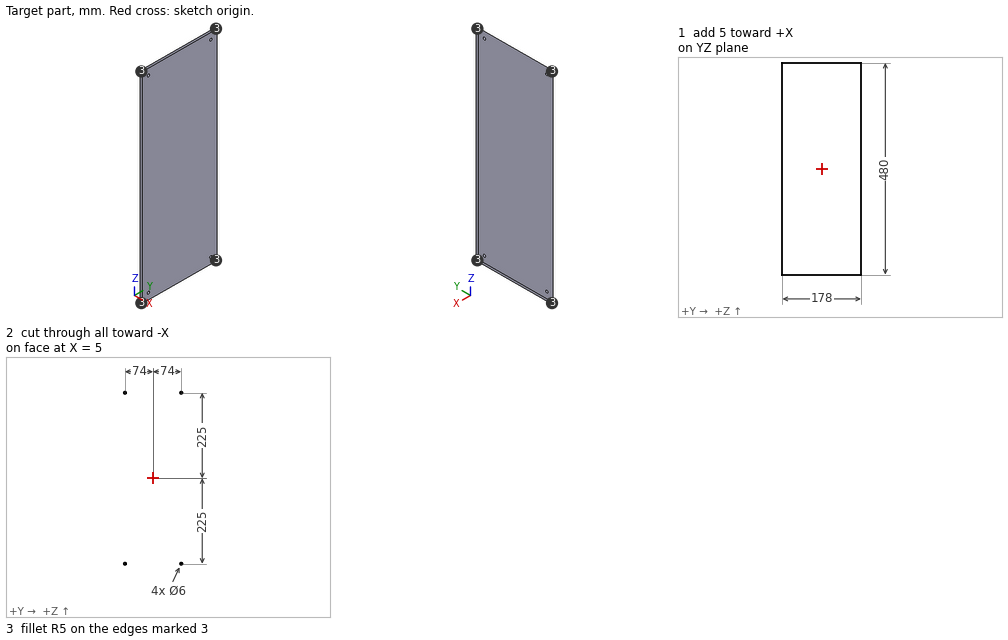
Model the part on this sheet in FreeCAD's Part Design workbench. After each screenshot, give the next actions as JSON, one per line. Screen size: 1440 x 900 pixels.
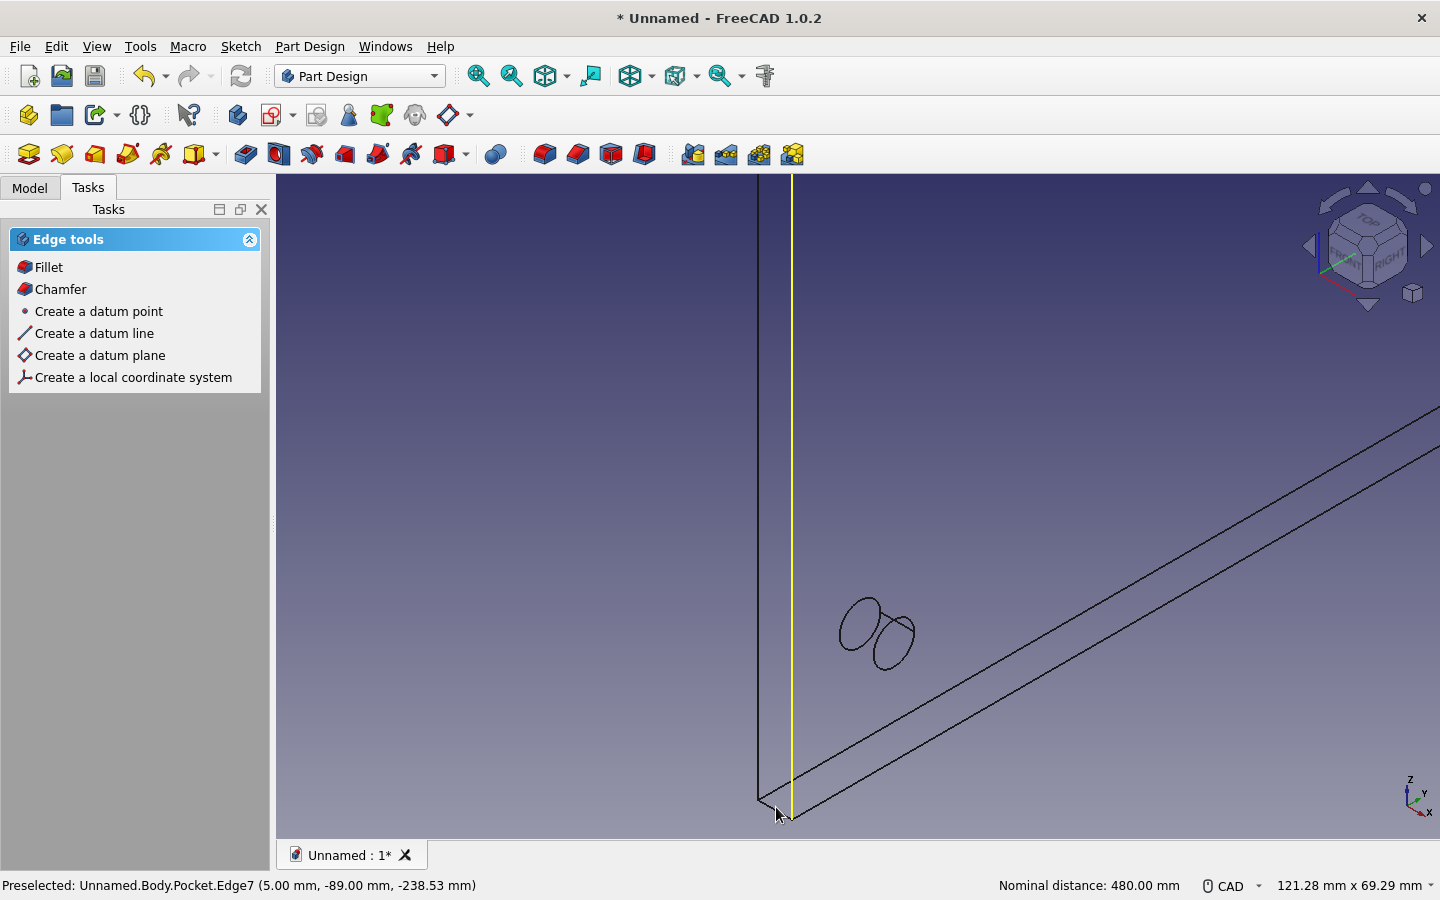
{"action": "left_click", "coordinate": [775, 809], "text": "ctrl"}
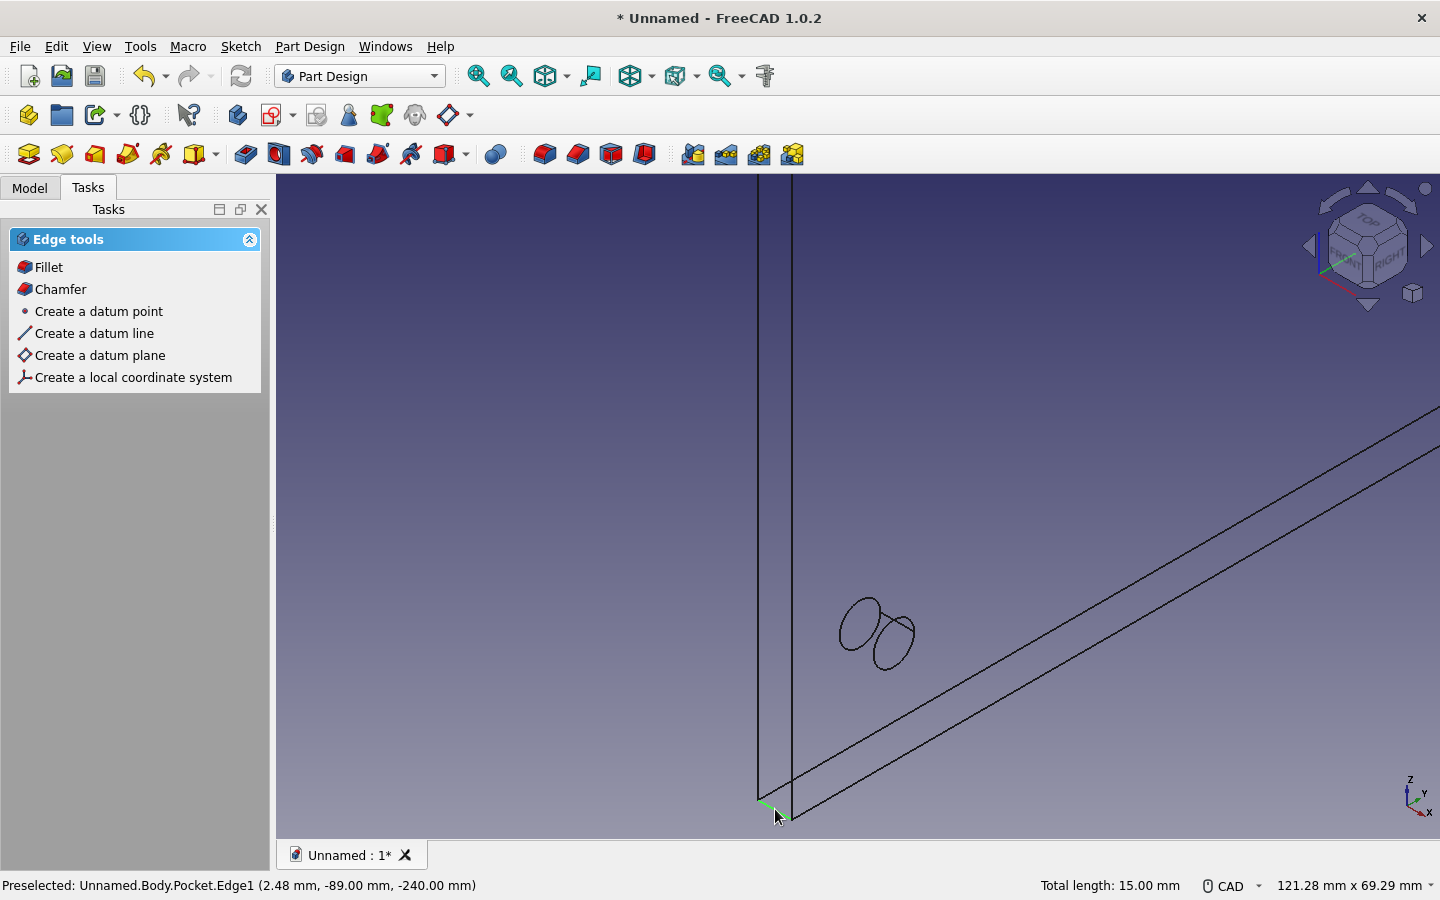
{"action": "left_click", "coordinate": [479, 76]}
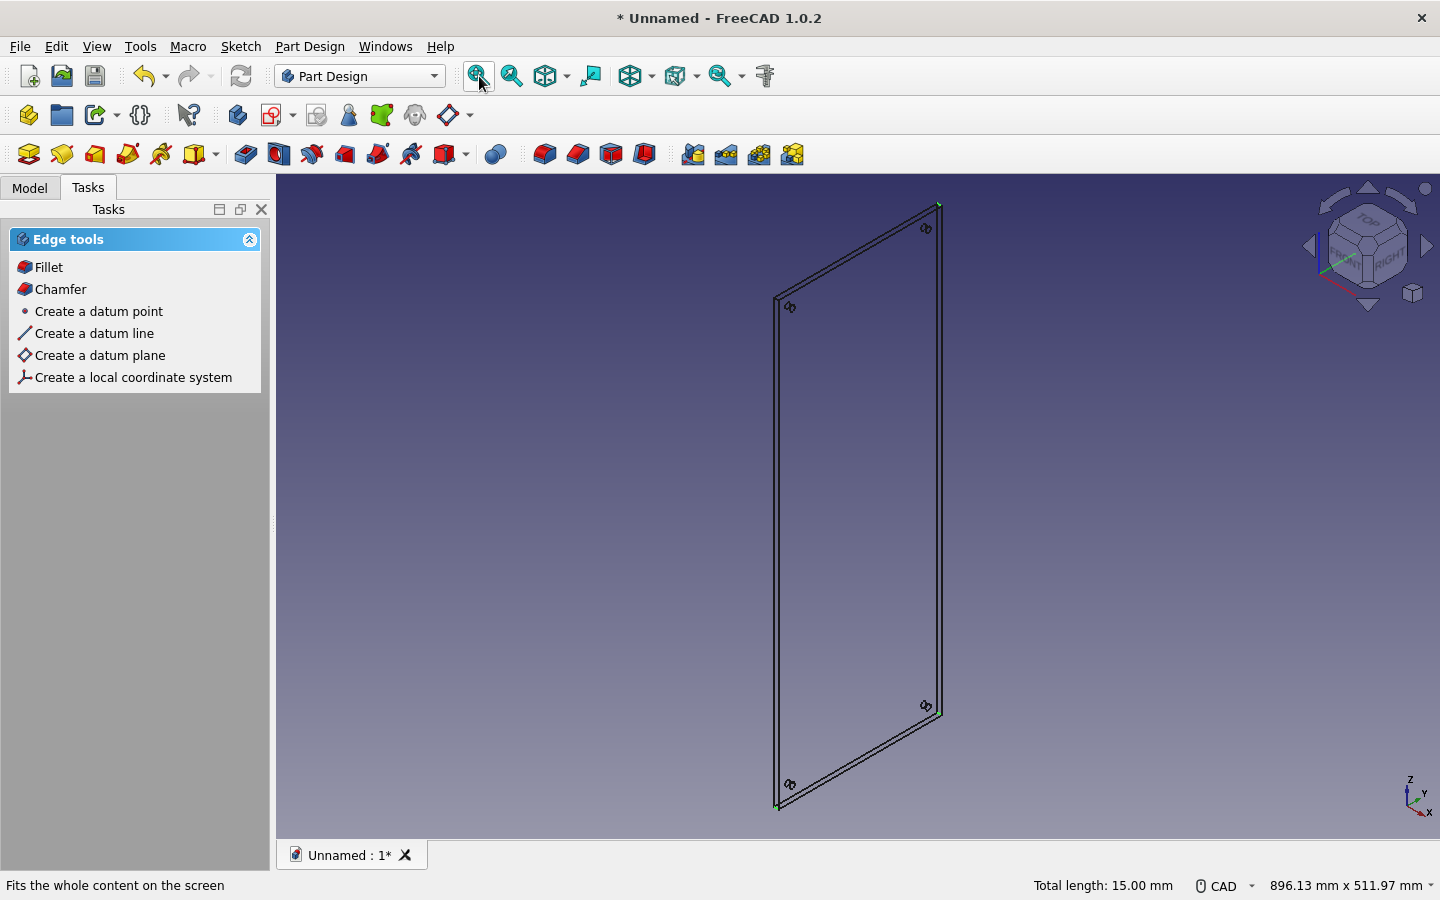
{"action": "key", "text": "2"}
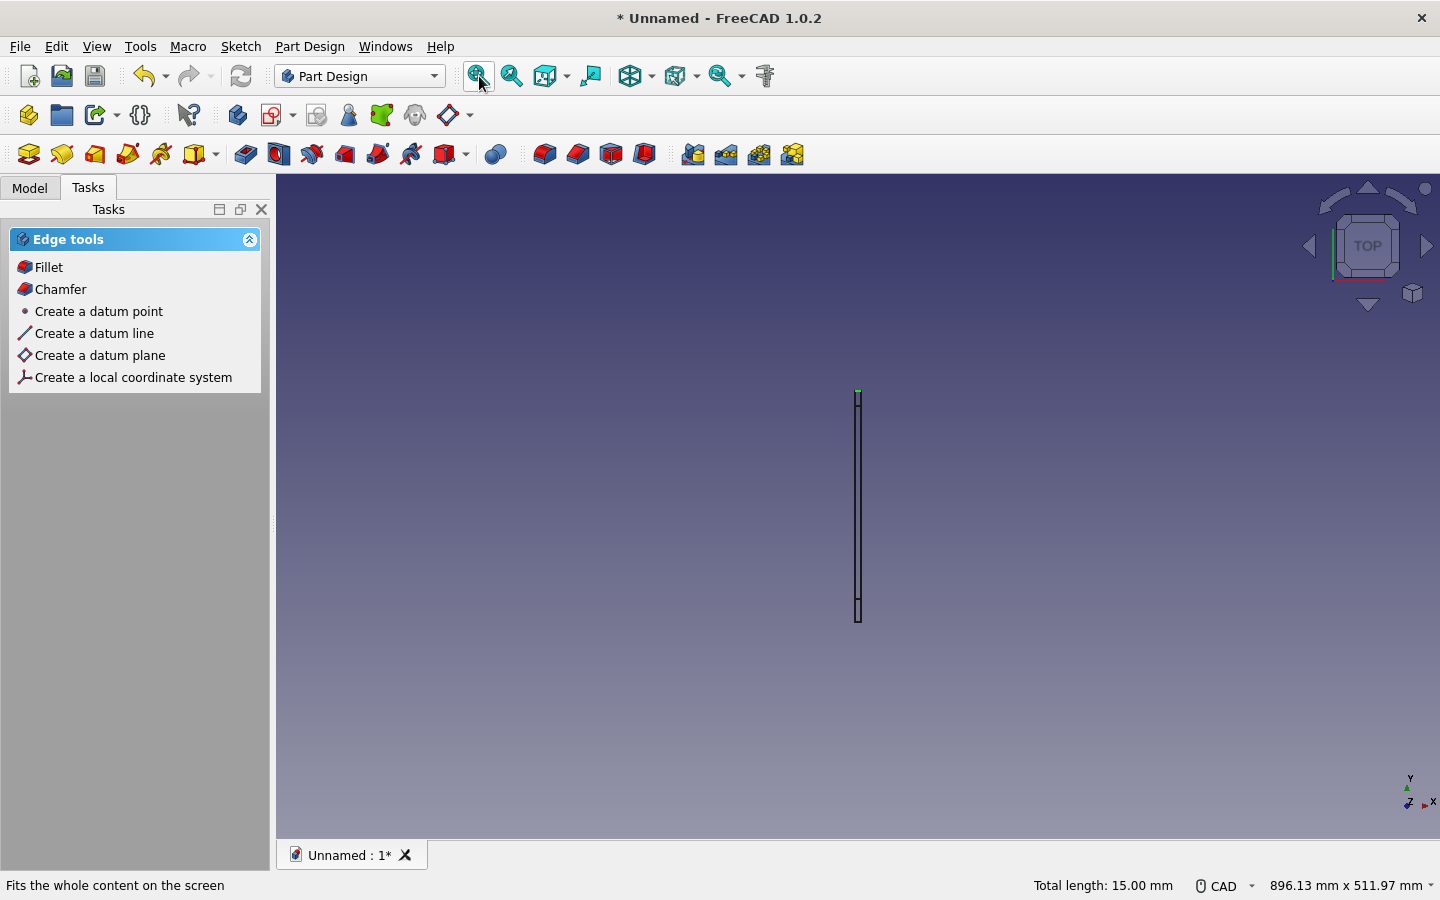
{"action": "left_click", "coordinate": [479, 76]}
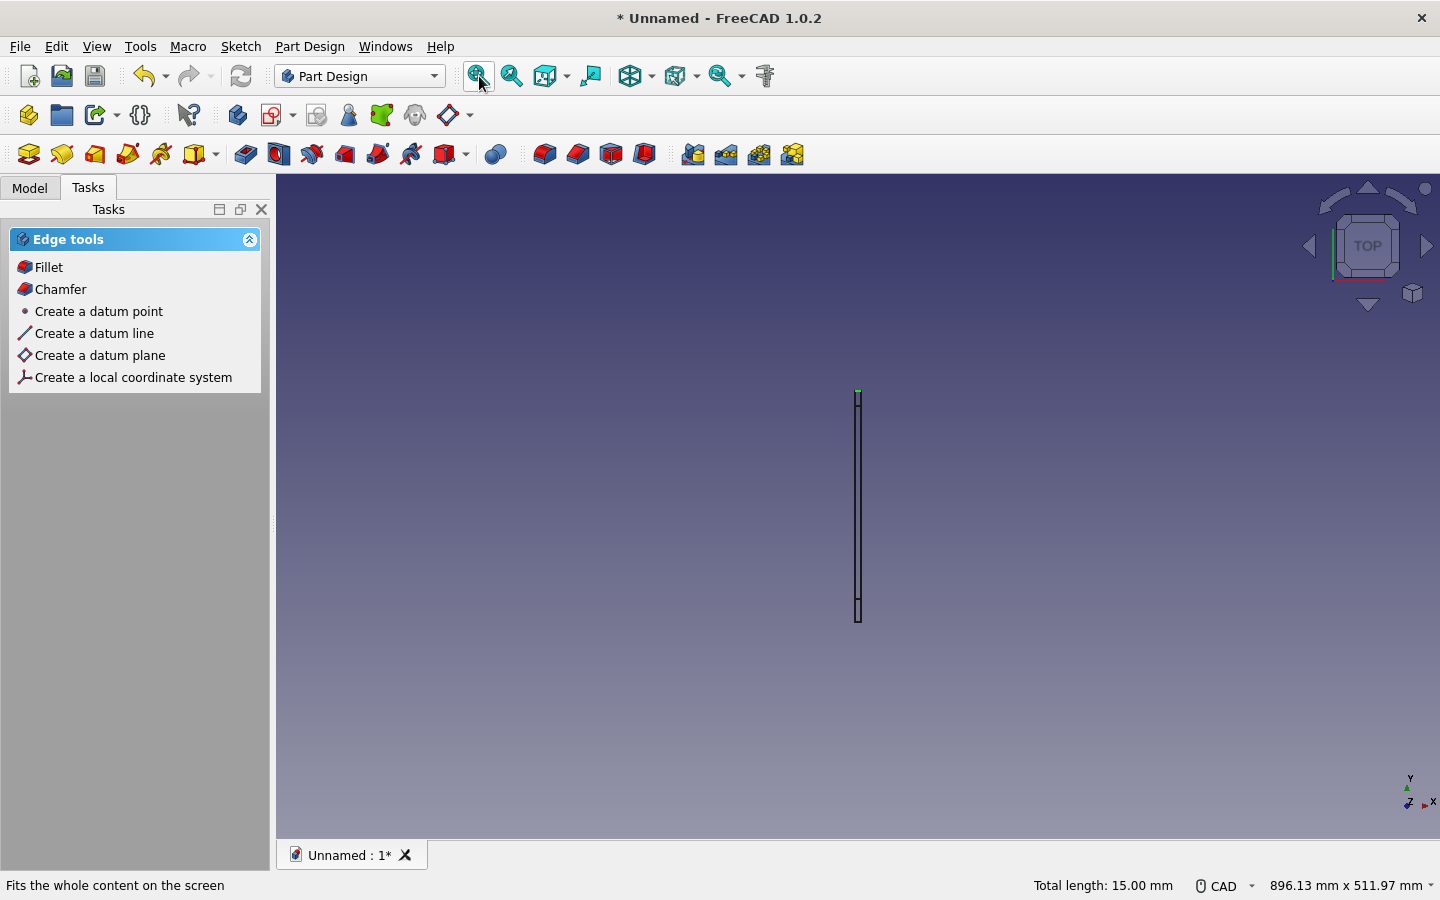
{"action": "scroll", "coordinate": [858, 621], "scroll_direction": "up", "scroll_amount": 10}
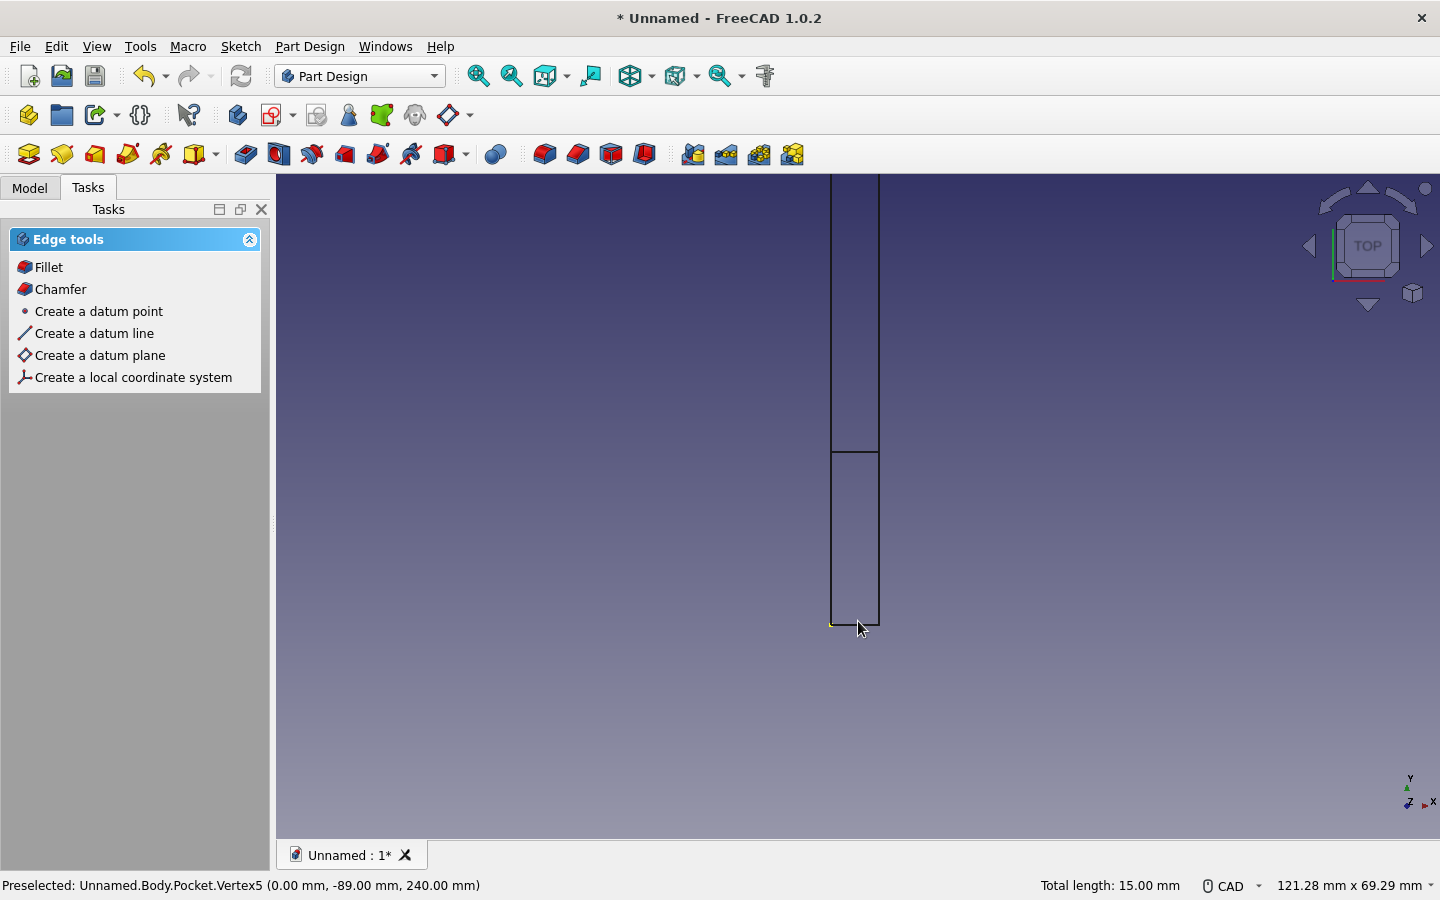
{"action": "left_click", "coordinate": [855, 624], "text": "ctrl"}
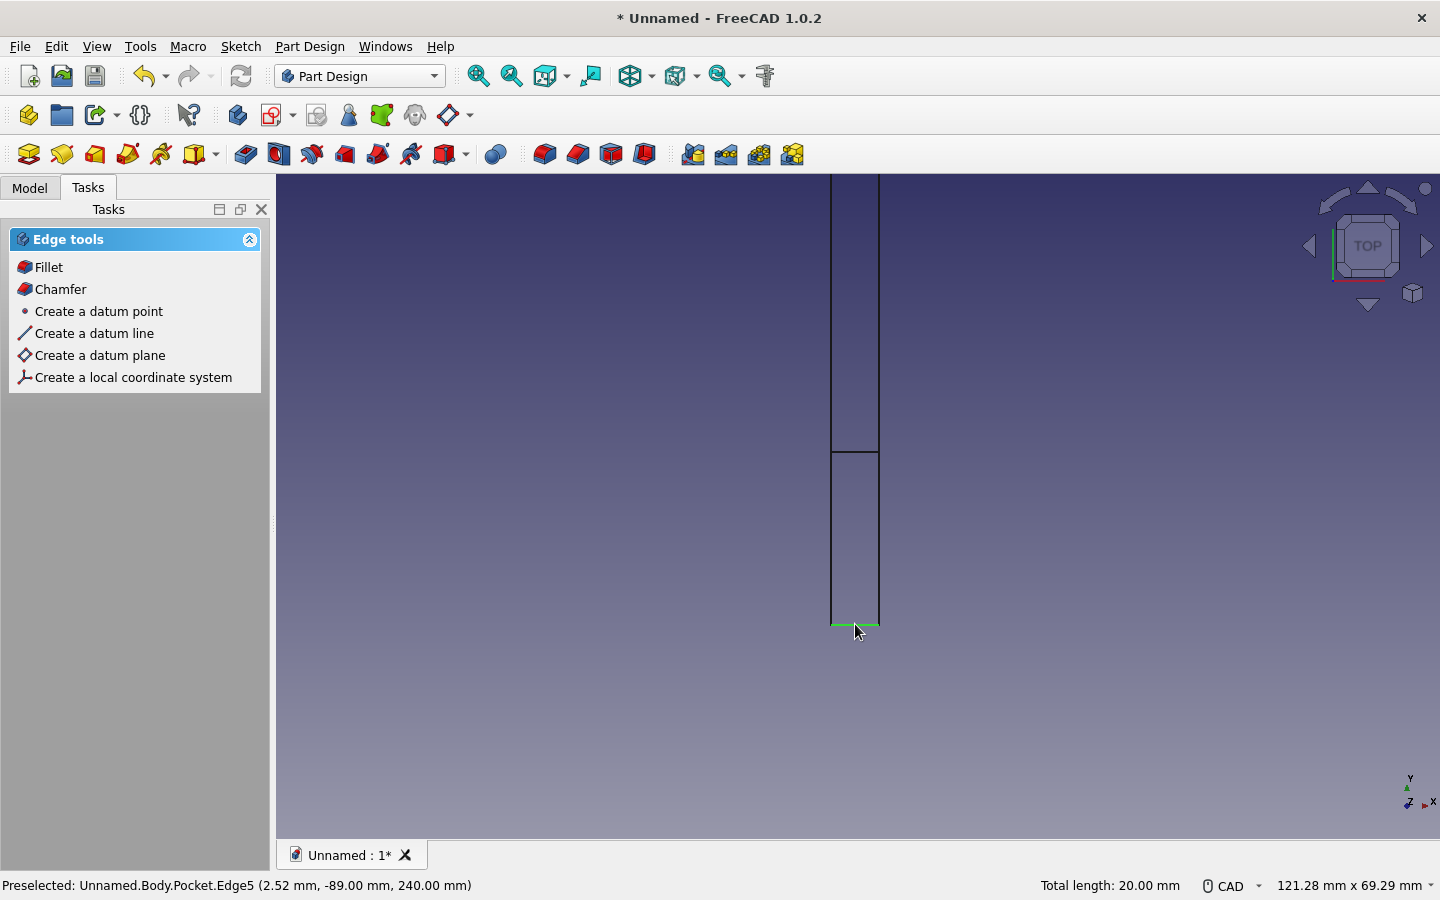
{"action": "key", "text": "v 1"}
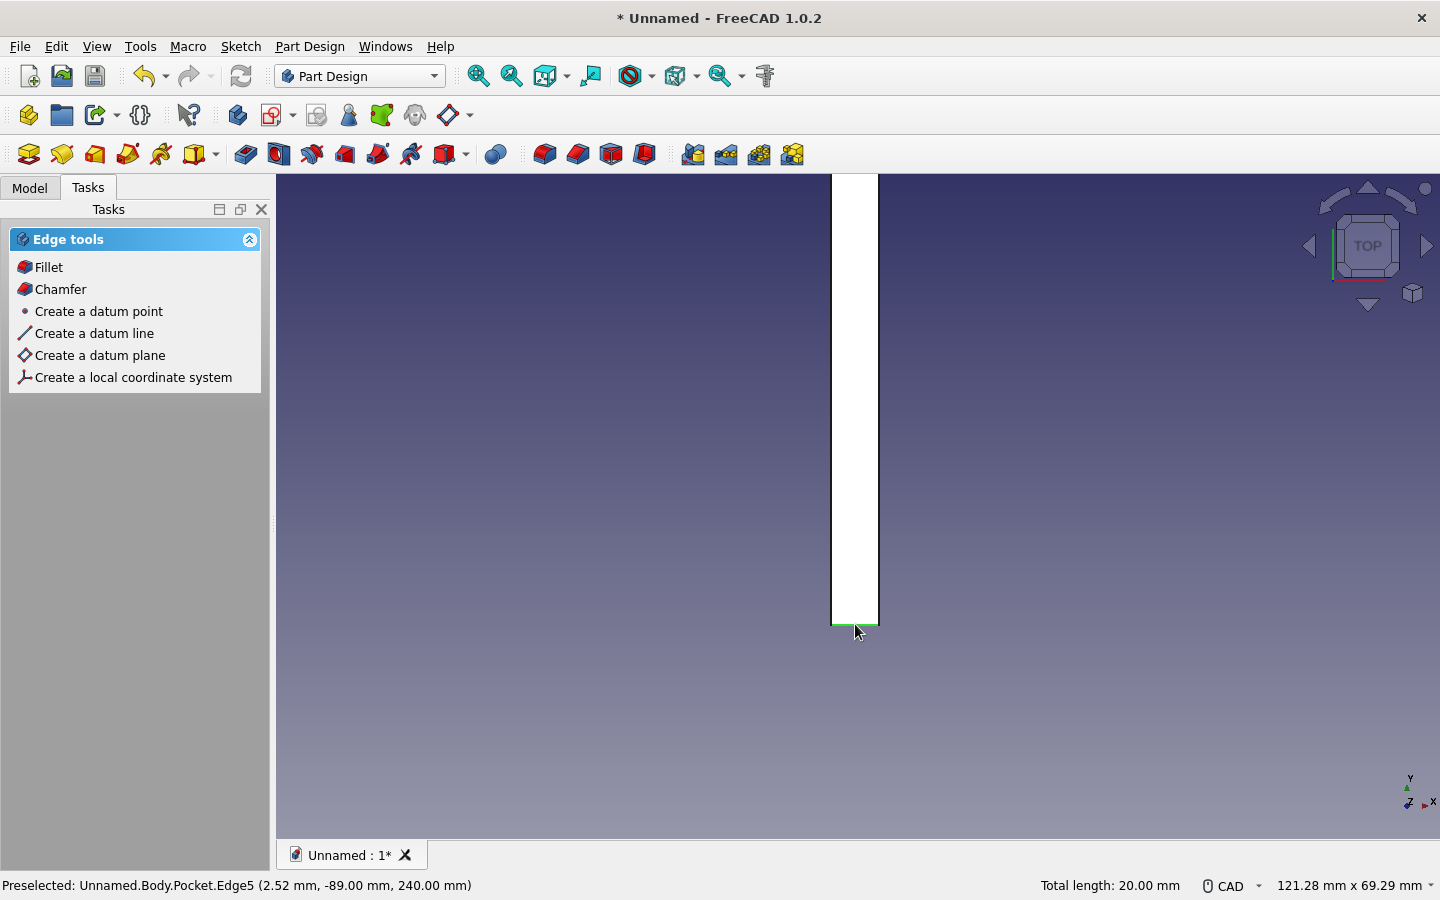
{"action": "left_click", "coordinate": [545, 154]}